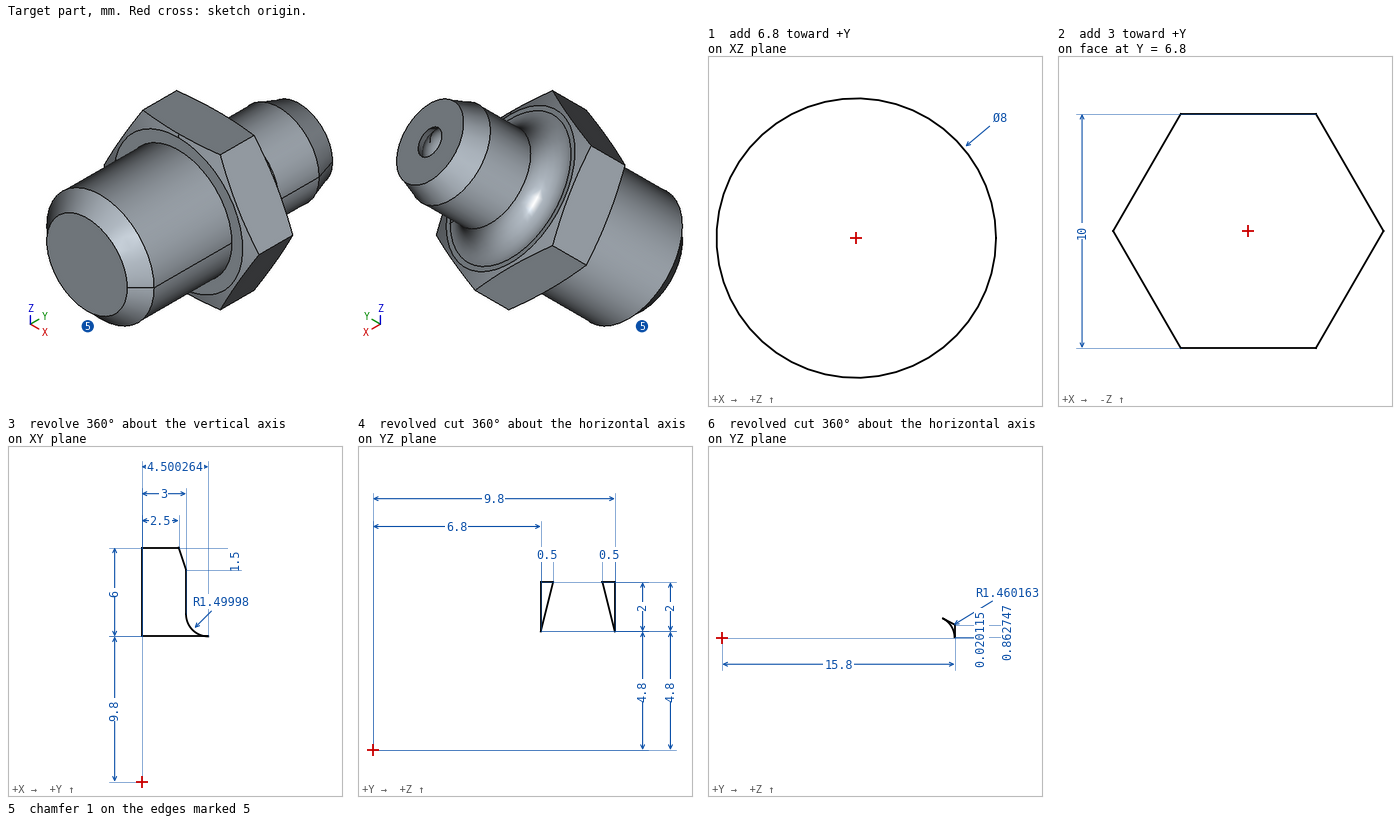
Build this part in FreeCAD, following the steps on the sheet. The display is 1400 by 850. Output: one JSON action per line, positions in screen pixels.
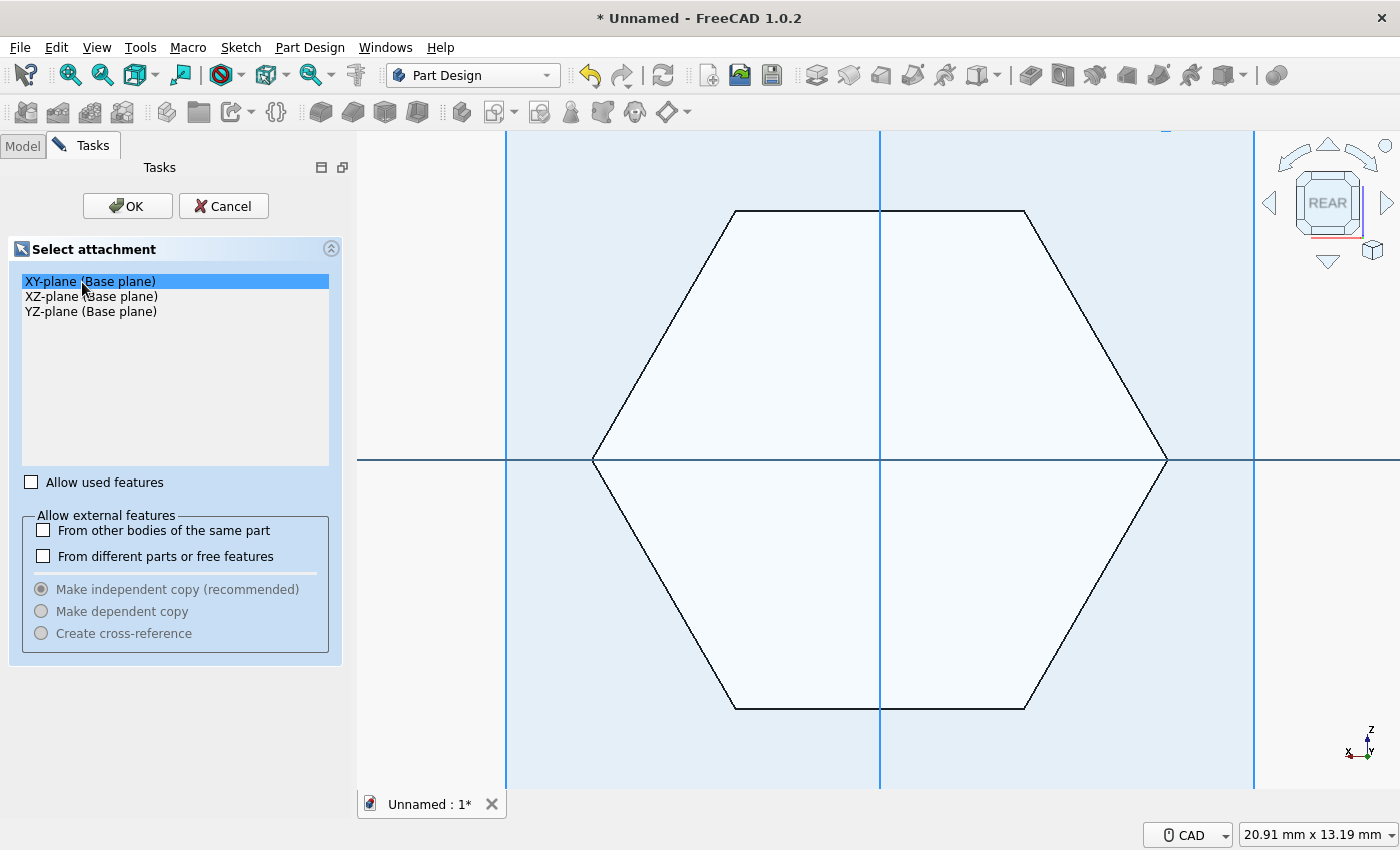
{"action": "left_click", "coordinate": [128, 206]}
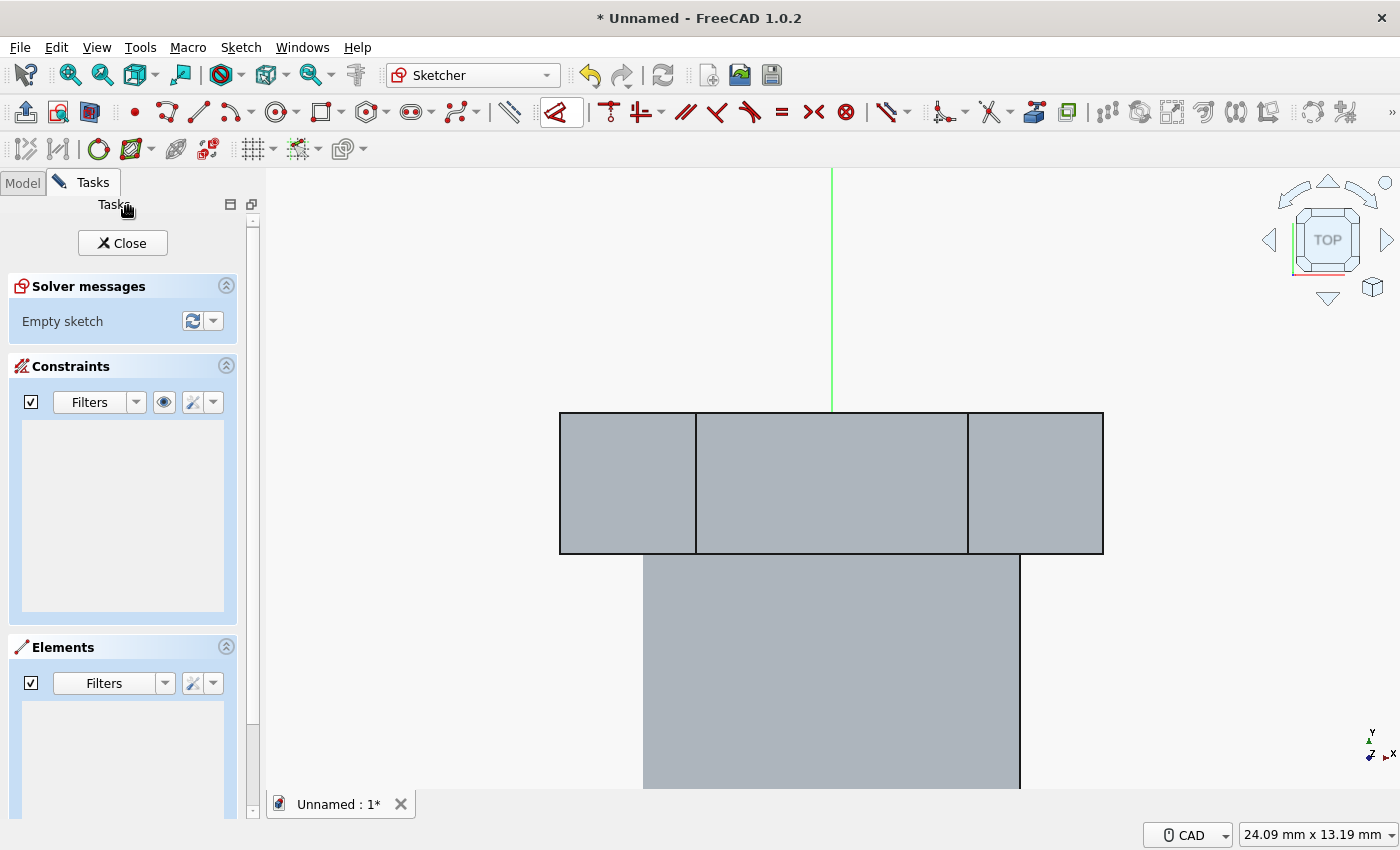
{"action": "left_click", "coordinate": [90, 112]}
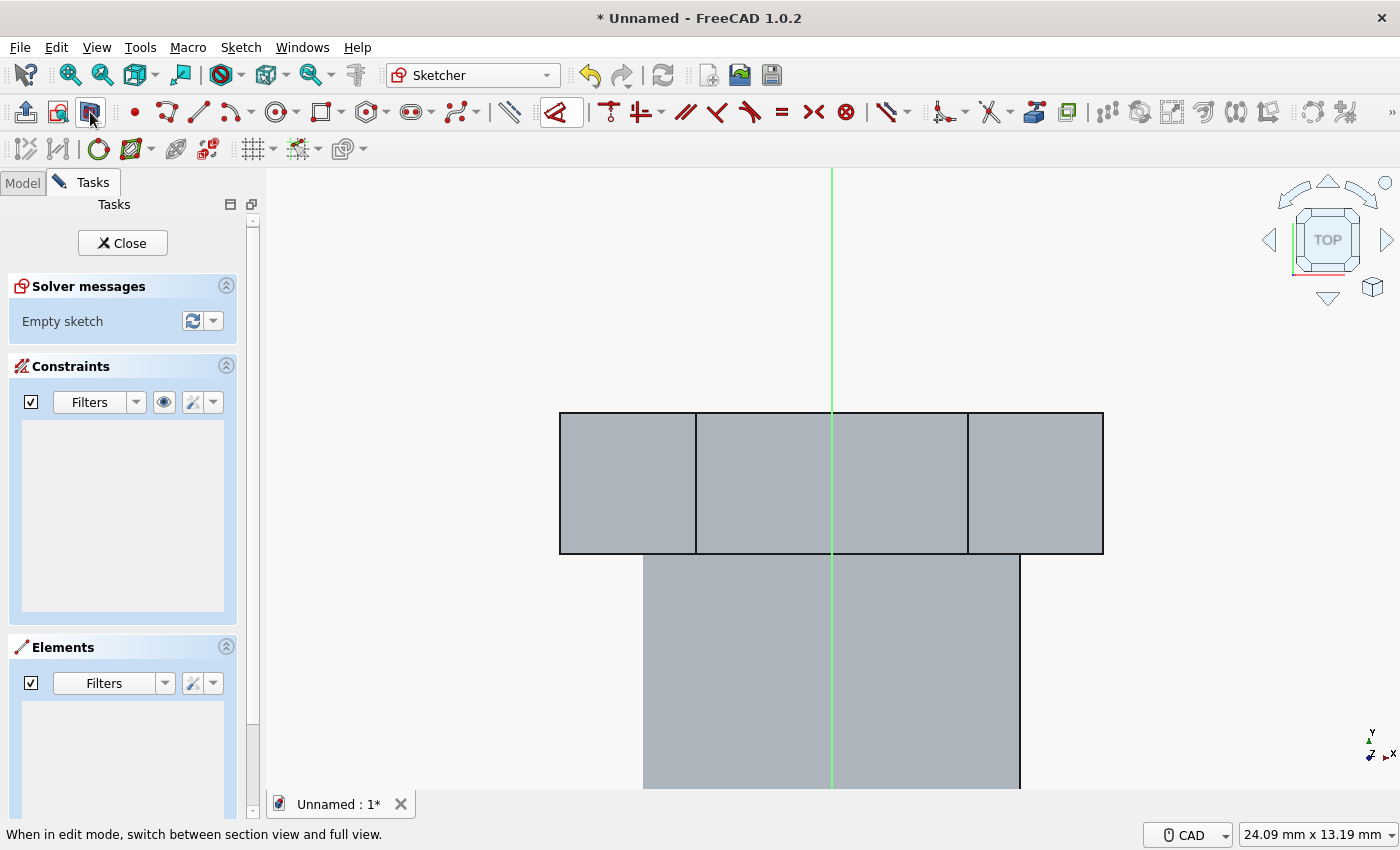
{"action": "scroll", "coordinate": [294, 761], "scroll_direction": "down", "scroll_amount": 1}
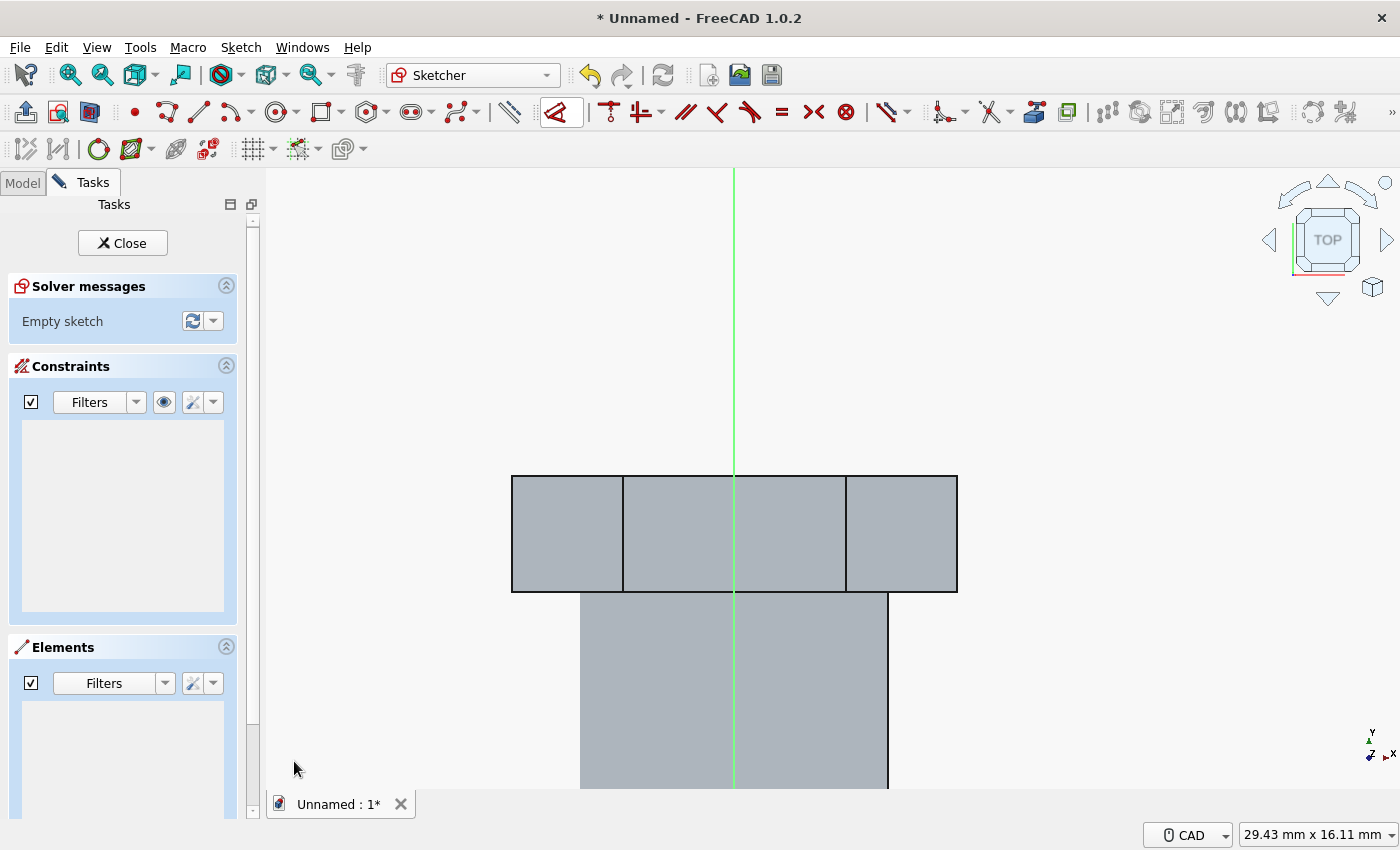
{"action": "scroll", "coordinate": [890, 217], "scroll_direction": "up", "scroll_amount": 3}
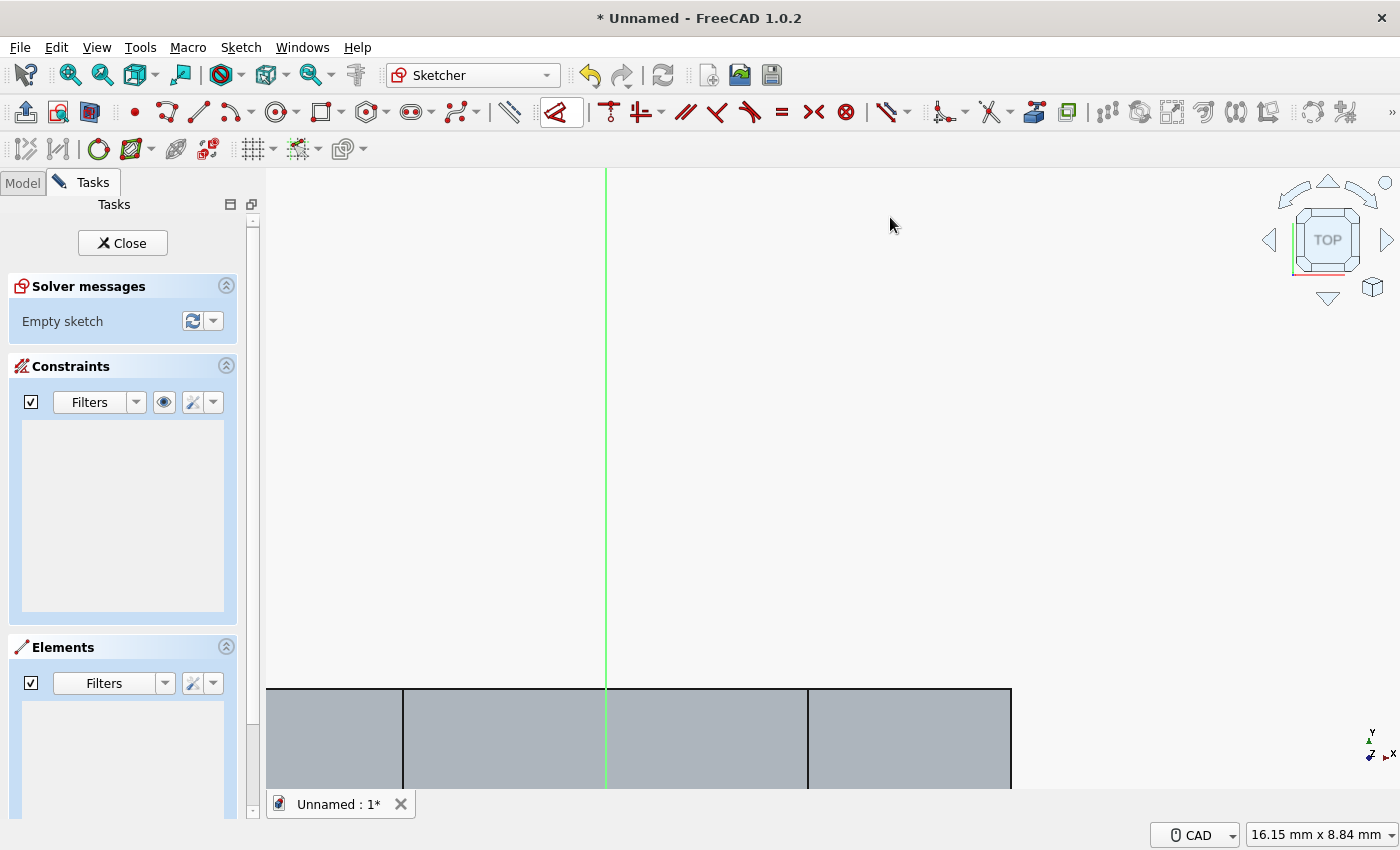
{"action": "left_click", "coordinate": [168, 112]}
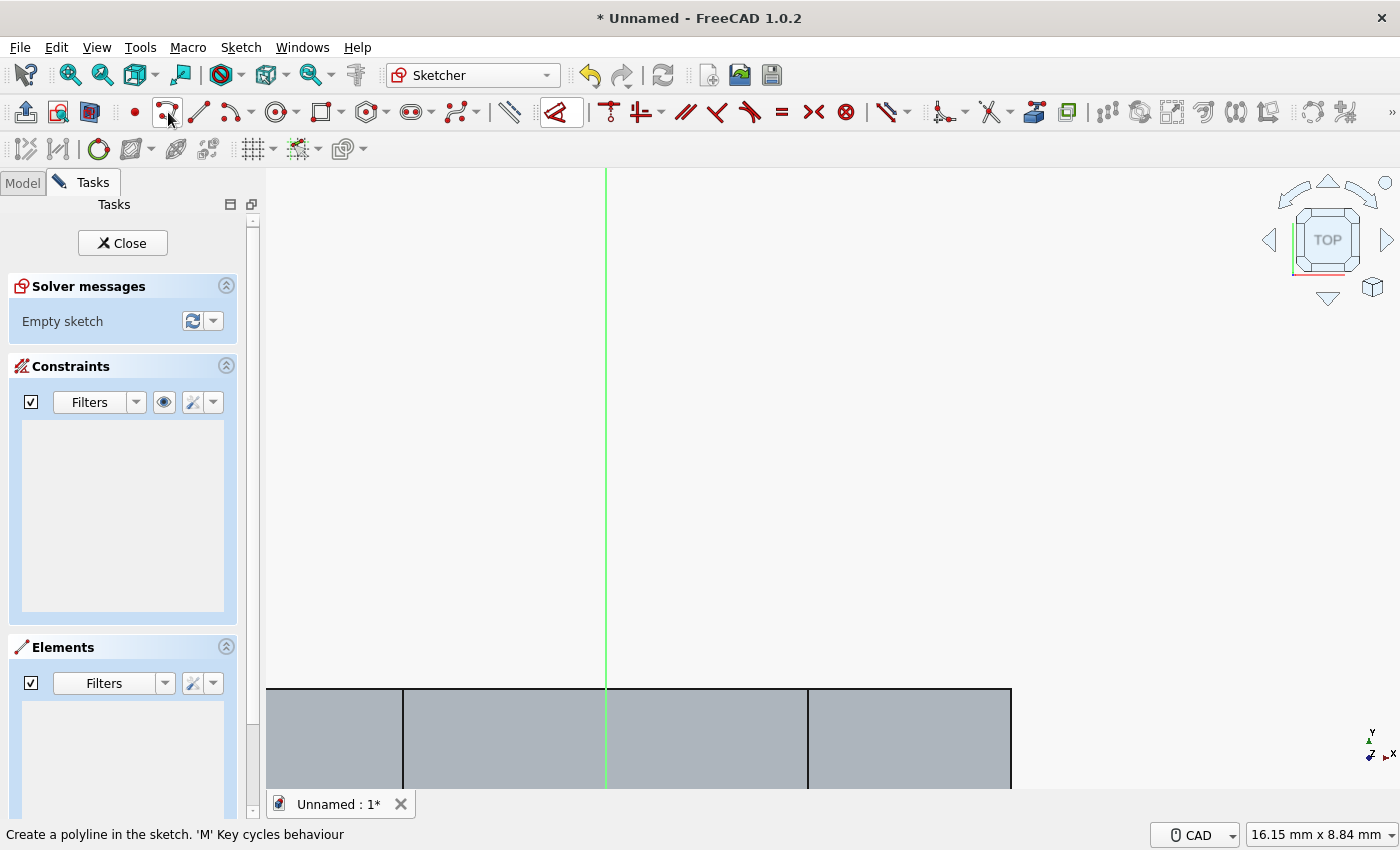
{"action": "left_click", "coordinate": [816, 583]}
{"action": "left_click", "coordinate": [816, 373]}
{"action": "left_click", "coordinate": [781, 267]}
{"action": "left_click", "coordinate": [606, 267]}
{"action": "left_click", "coordinate": [615, 689]}
{"action": "left_click", "coordinate": [922, 689]}
{"action": "right_click", "coordinate": [922, 689]}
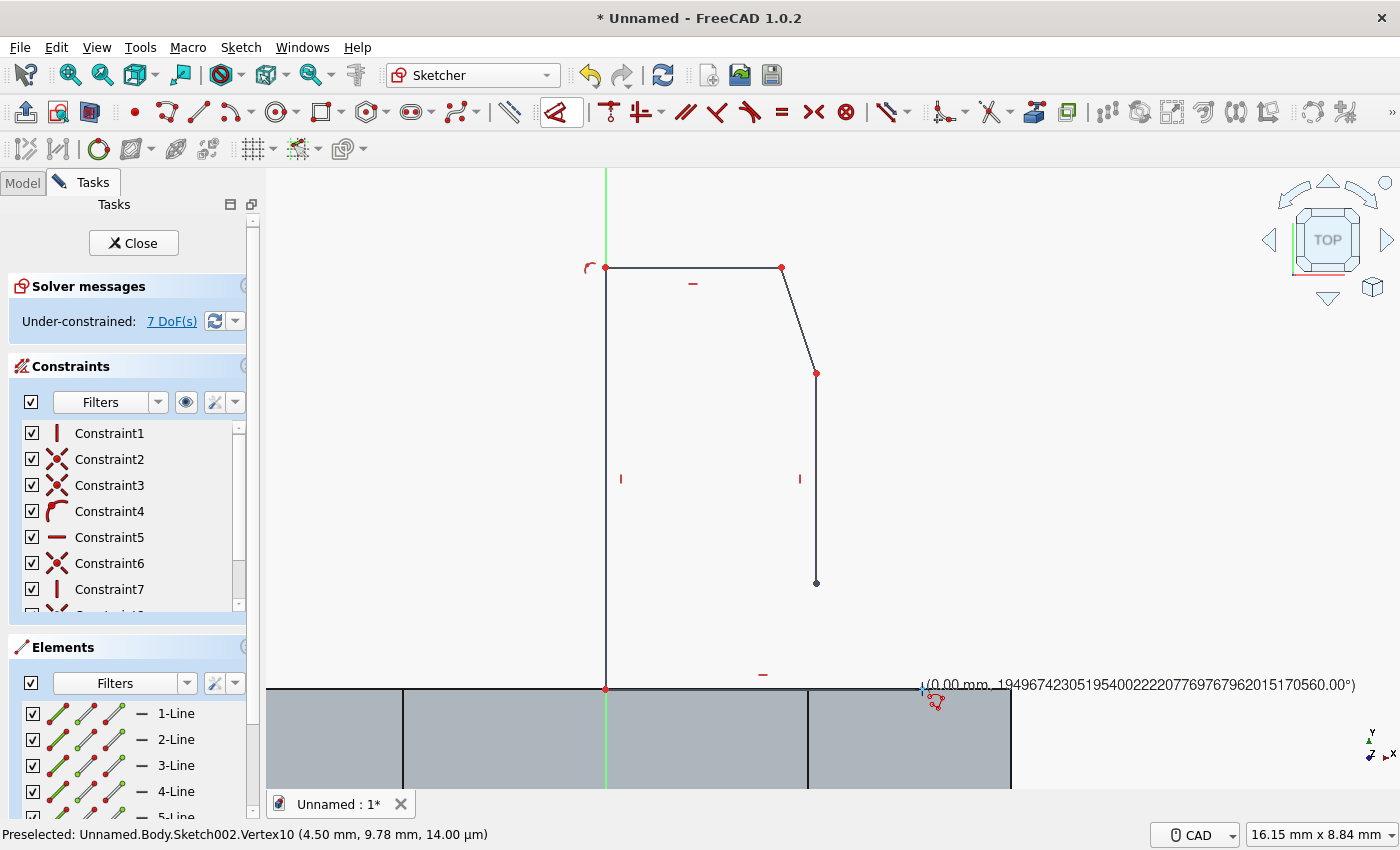
{"action": "key", "text": "g 3 a"}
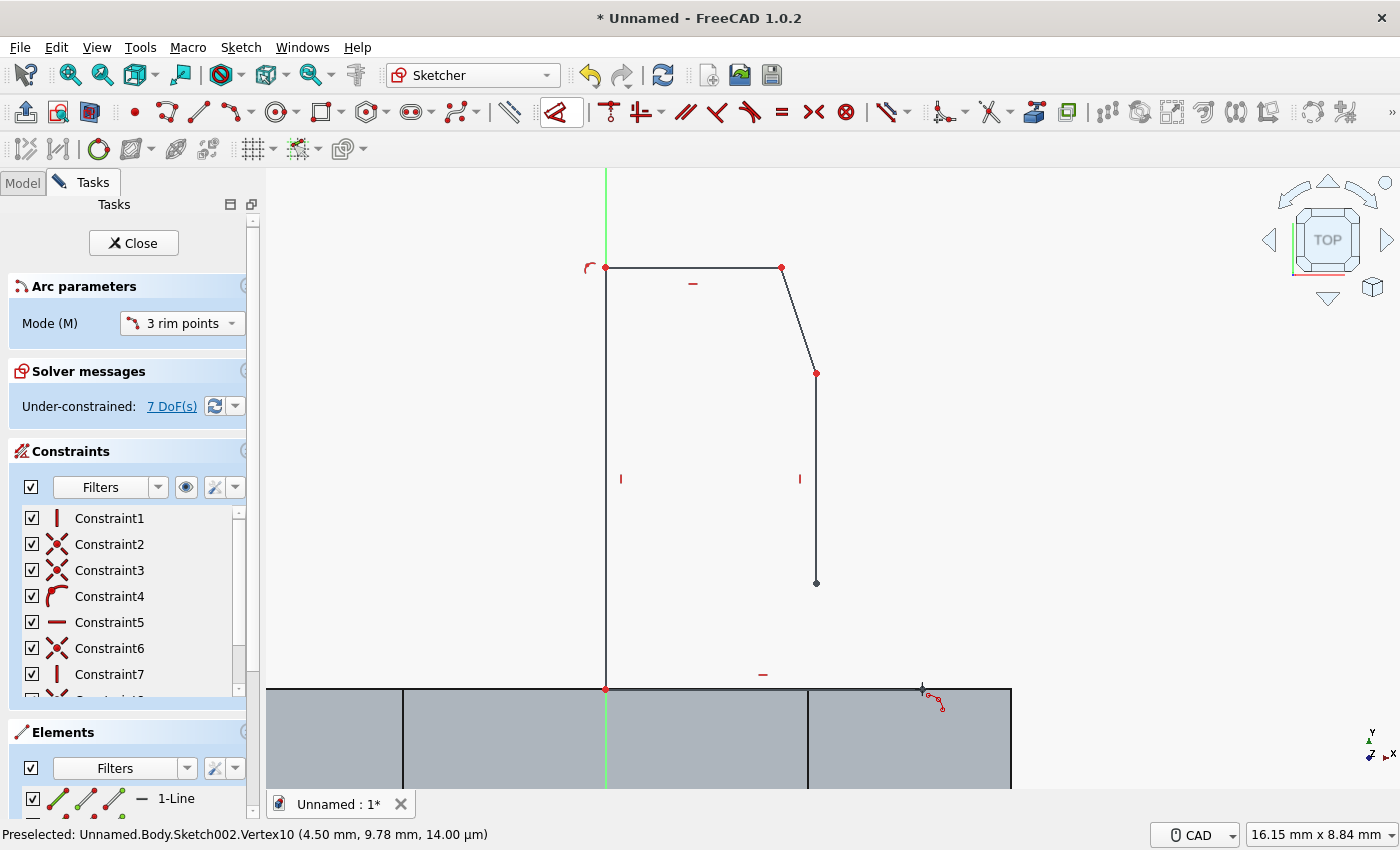
{"action": "left_click", "coordinate": [922, 690]}
{"action": "left_click", "coordinate": [816, 584]}
{"action": "left_click", "coordinate": [847, 658]}
{"action": "key", "text": "Escape"}